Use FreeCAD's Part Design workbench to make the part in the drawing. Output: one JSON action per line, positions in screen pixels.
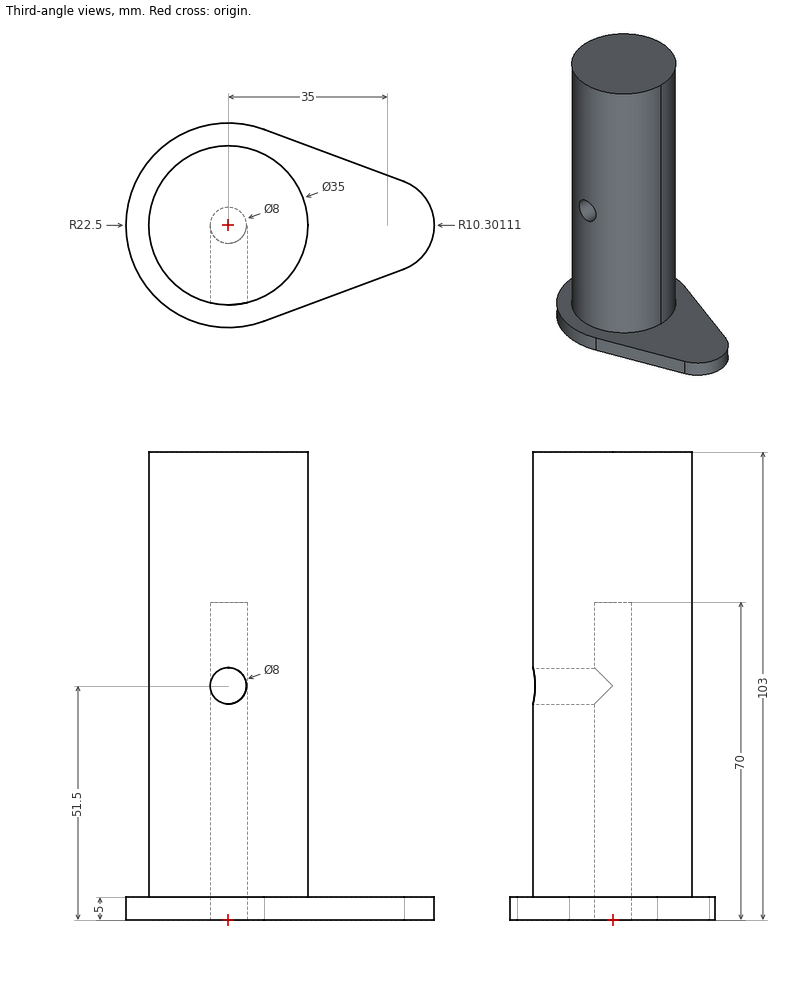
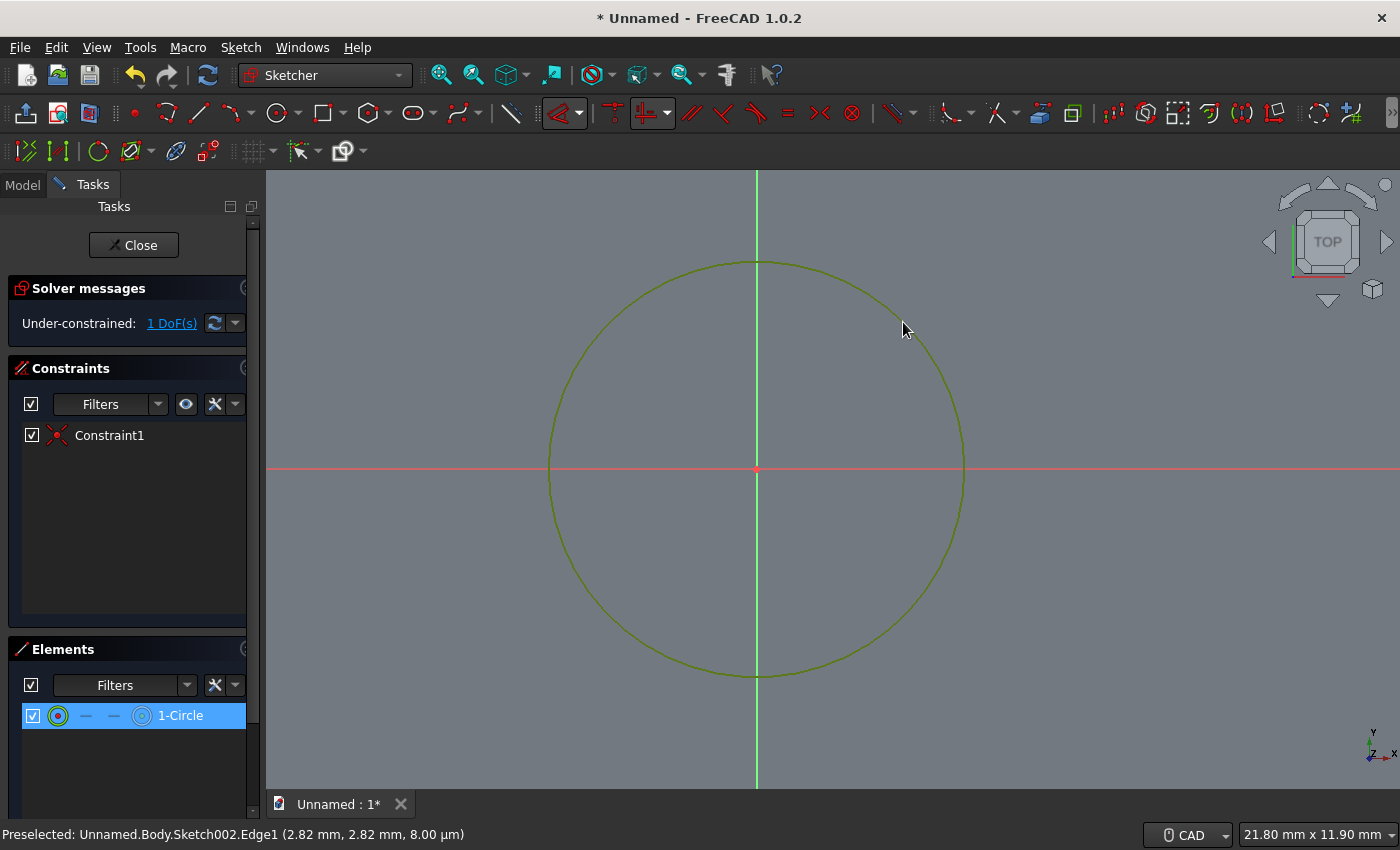
{"action": "left_click", "coordinate": [582, 114]}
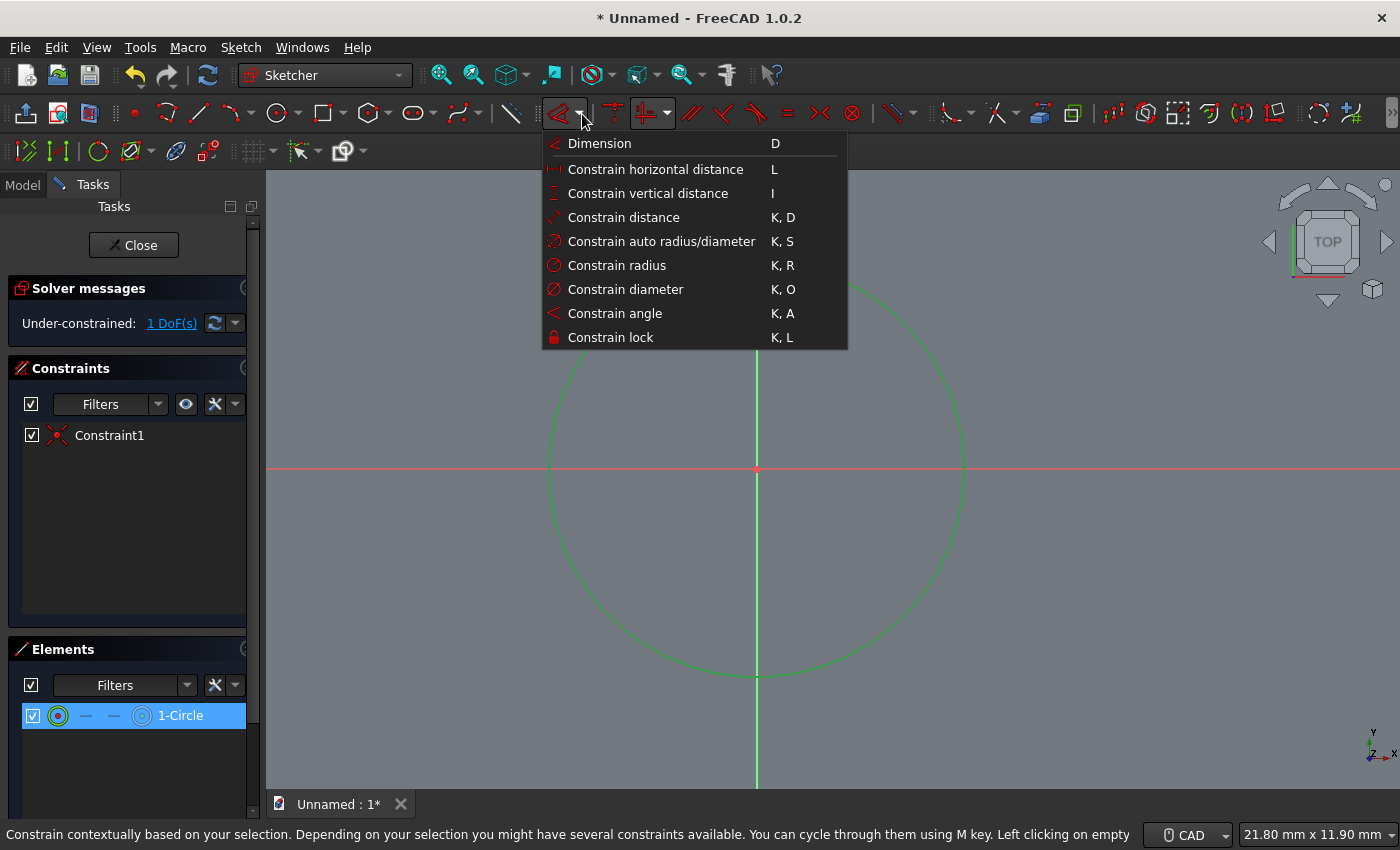
{"action": "left_click", "coordinate": [695, 289]}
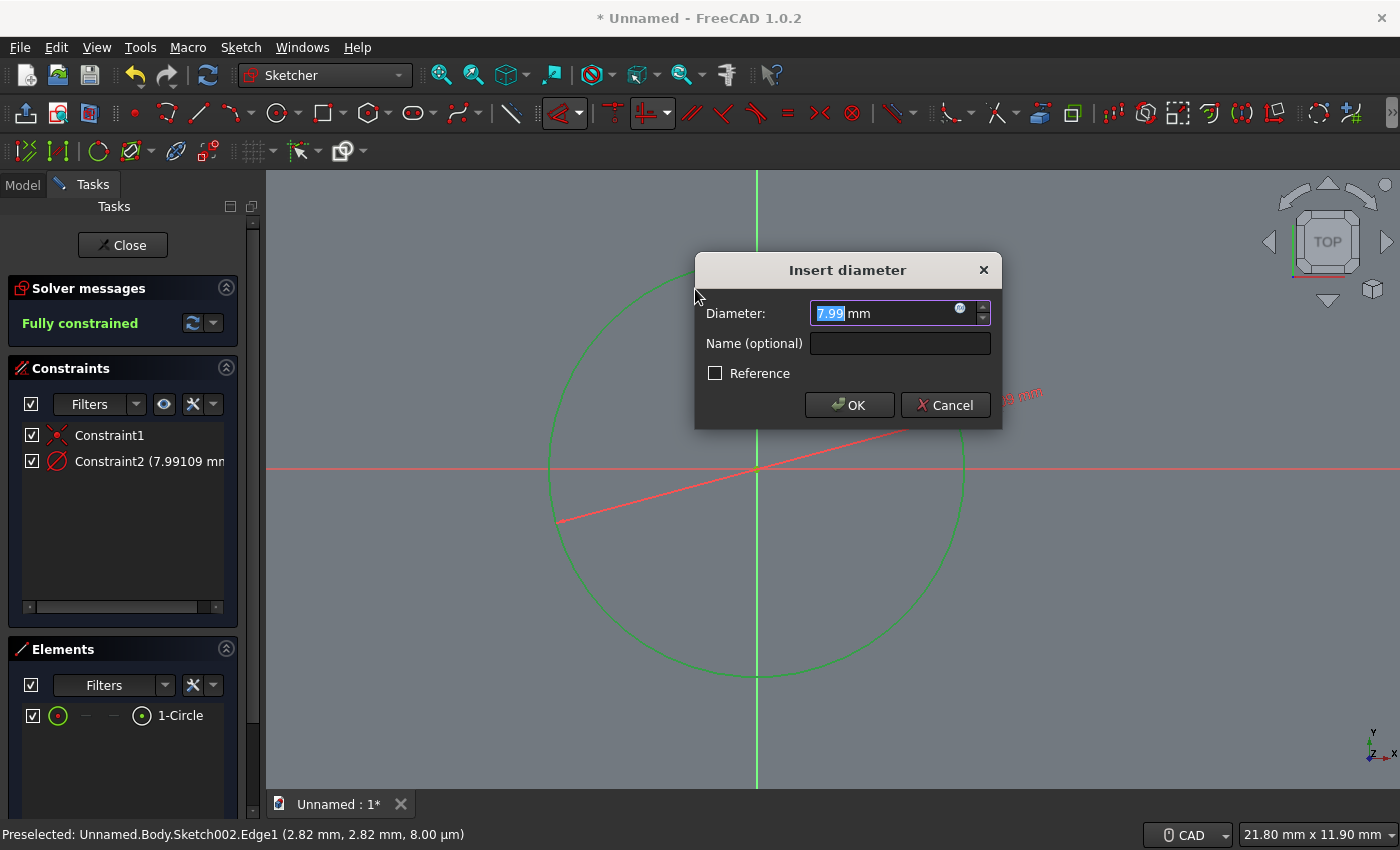
{"action": "type", "text": "8"}
{"action": "key", "text": "Return"}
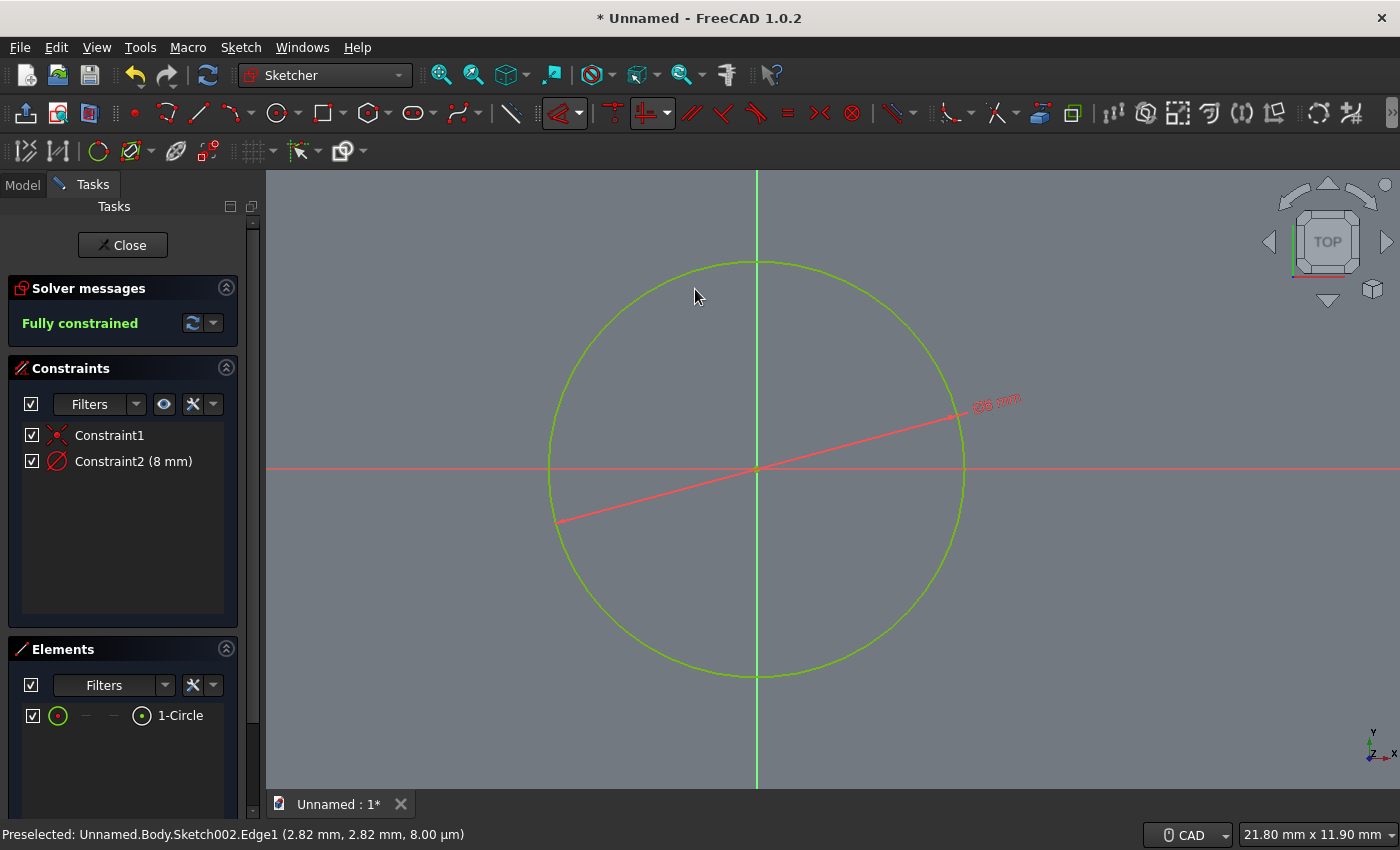
{"action": "left_click", "coordinate": [123, 245]}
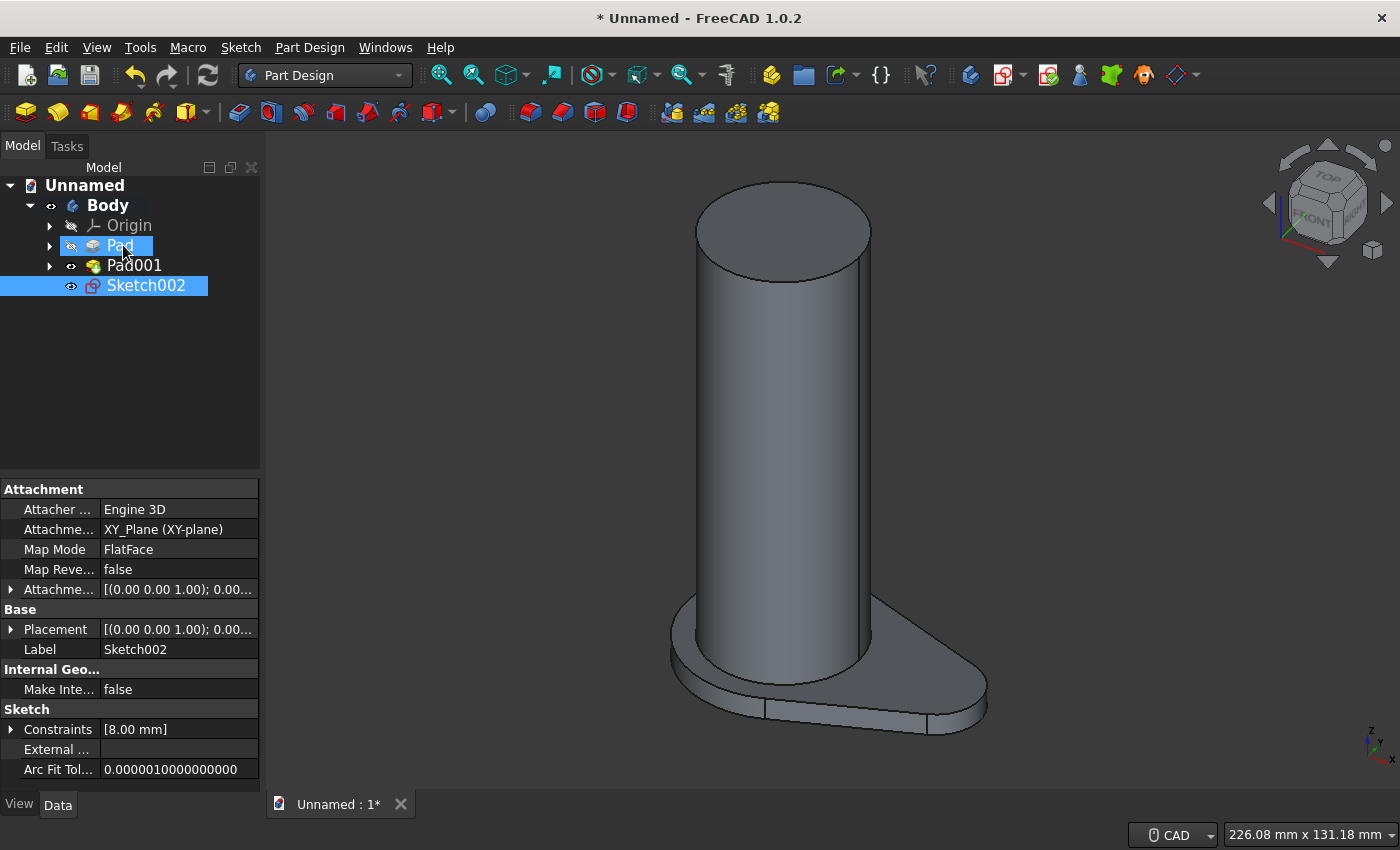
{"action": "left_click", "coordinate": [240, 112]}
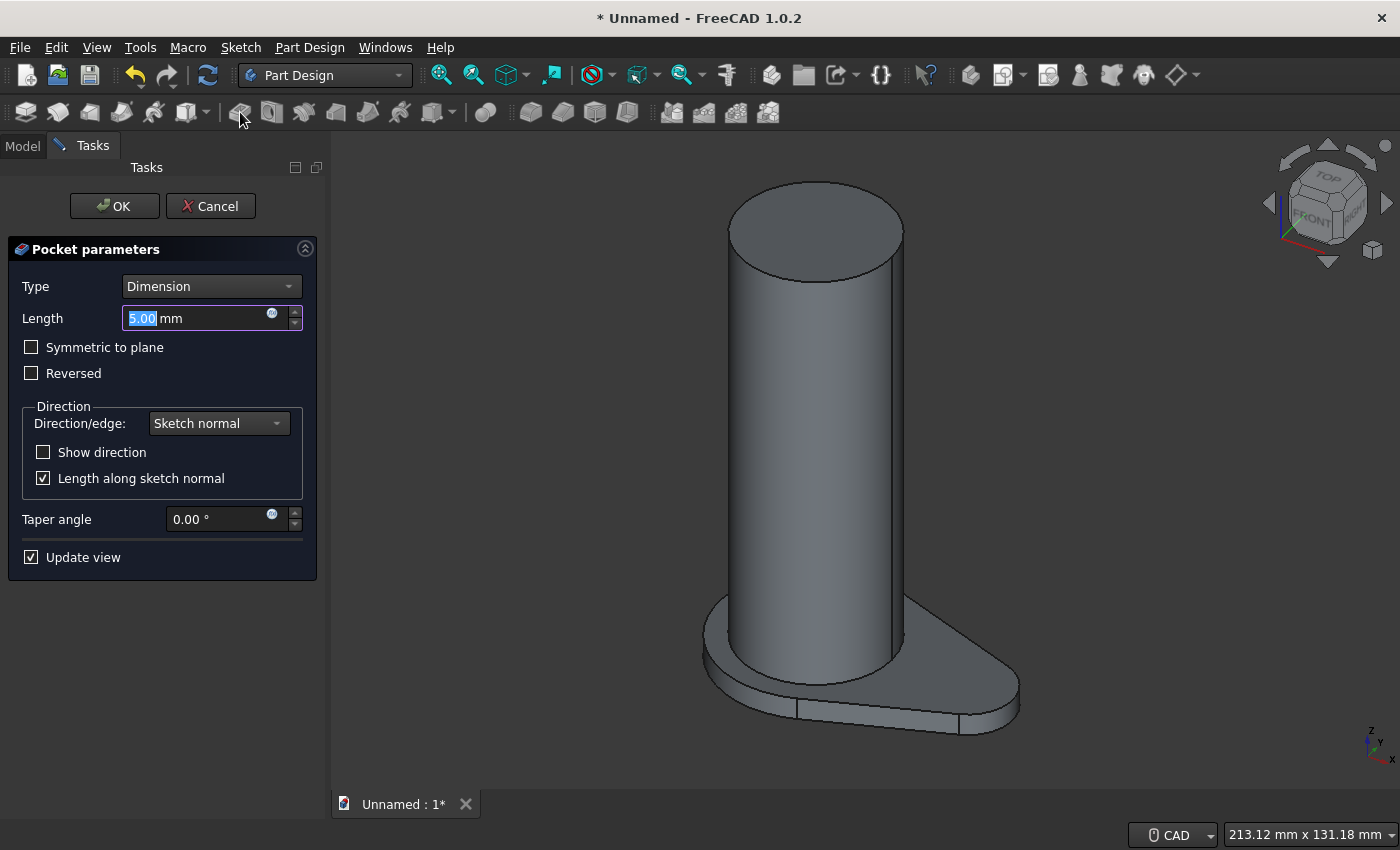
{"action": "type", "text": "70"}
{"action": "key", "text": "Tab"}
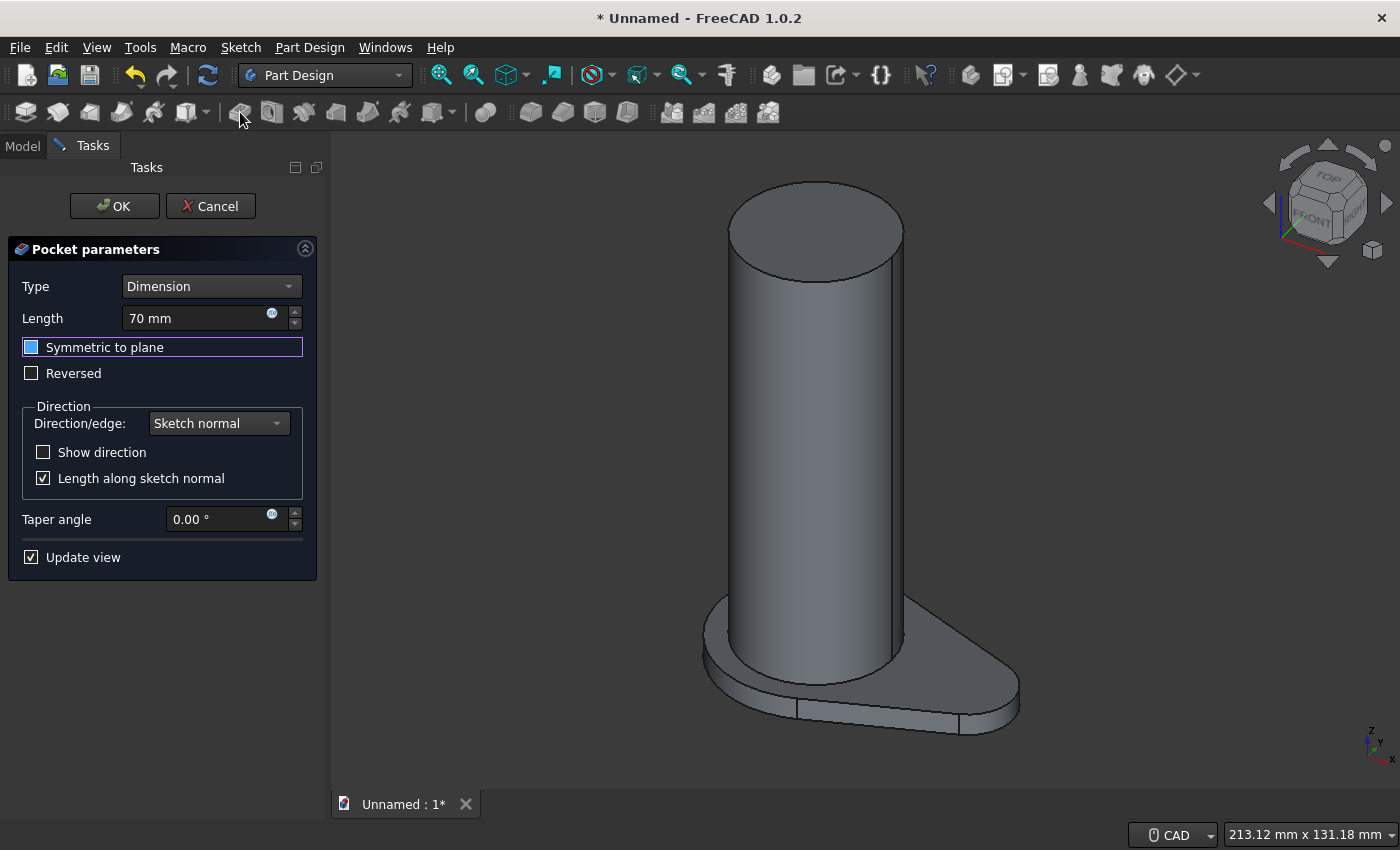
{"action": "left_click", "coordinate": [30, 373]}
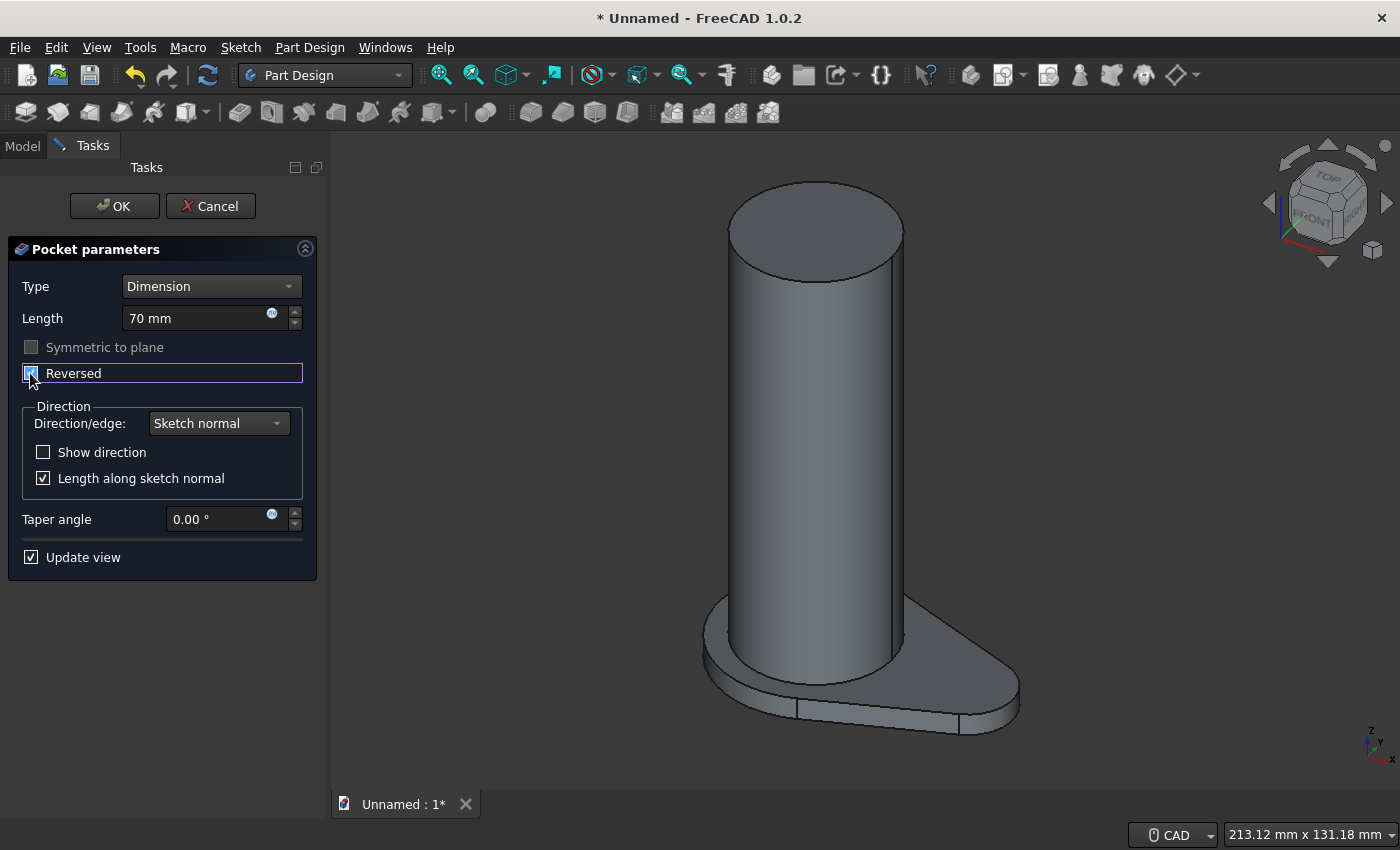
{"action": "left_click", "coordinate": [115, 206]}